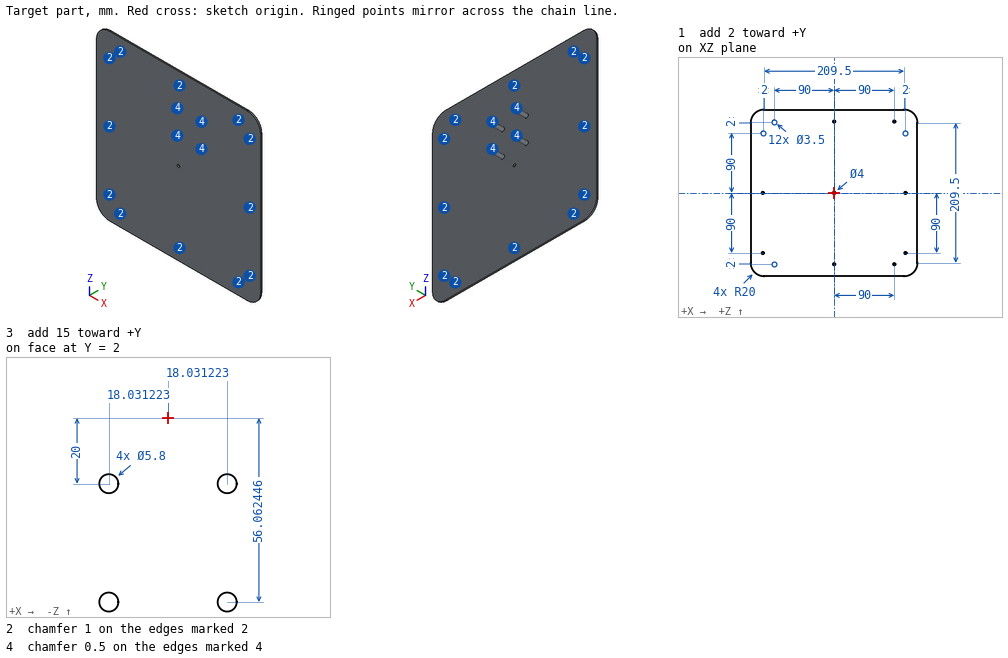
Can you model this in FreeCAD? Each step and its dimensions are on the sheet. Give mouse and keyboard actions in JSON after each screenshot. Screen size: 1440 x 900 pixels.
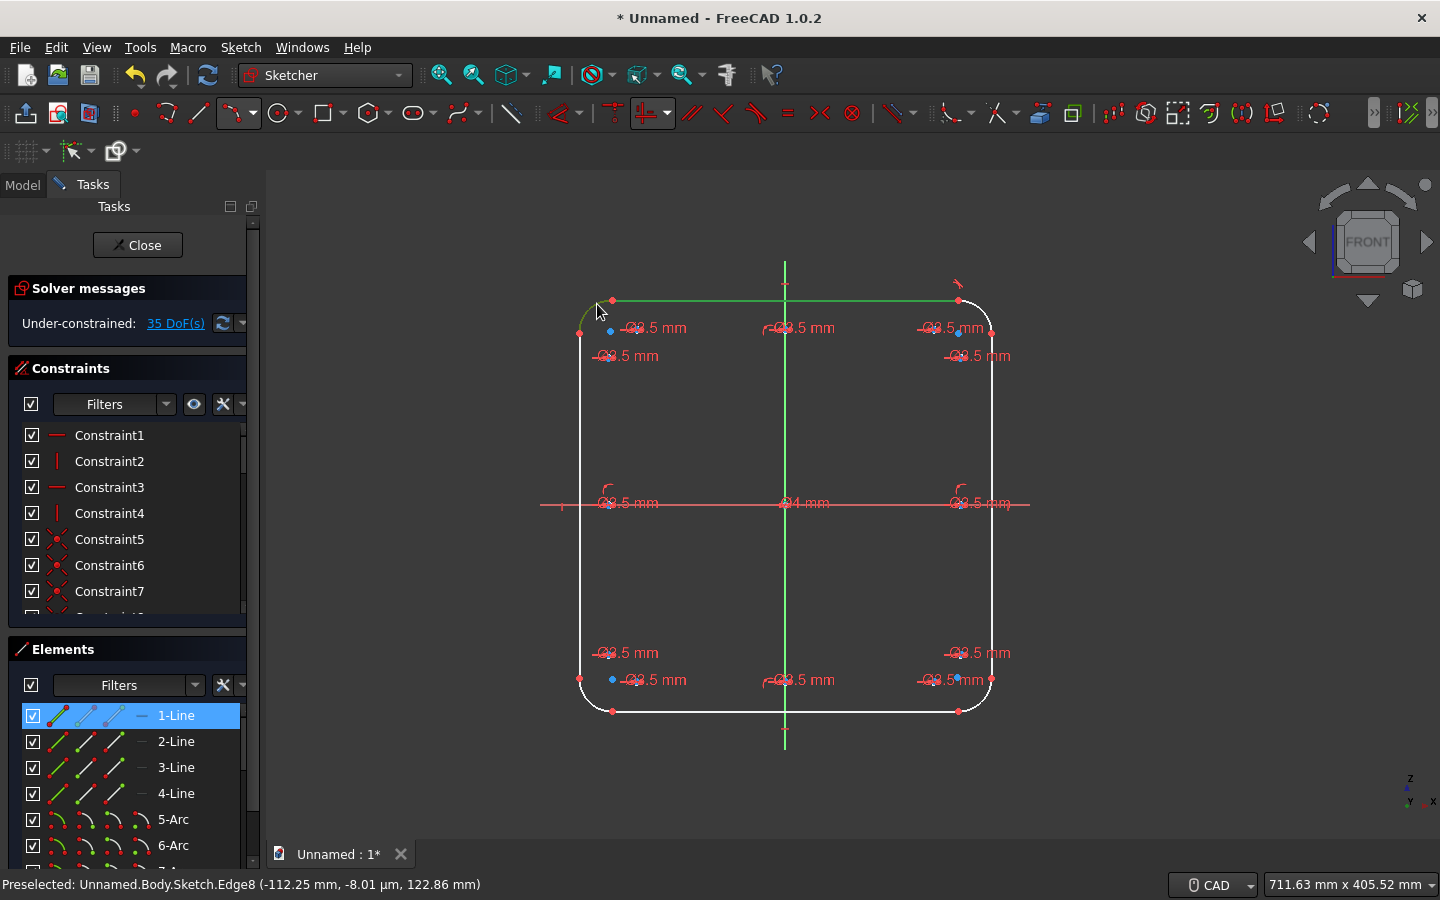
{"action": "key", "text": "t"}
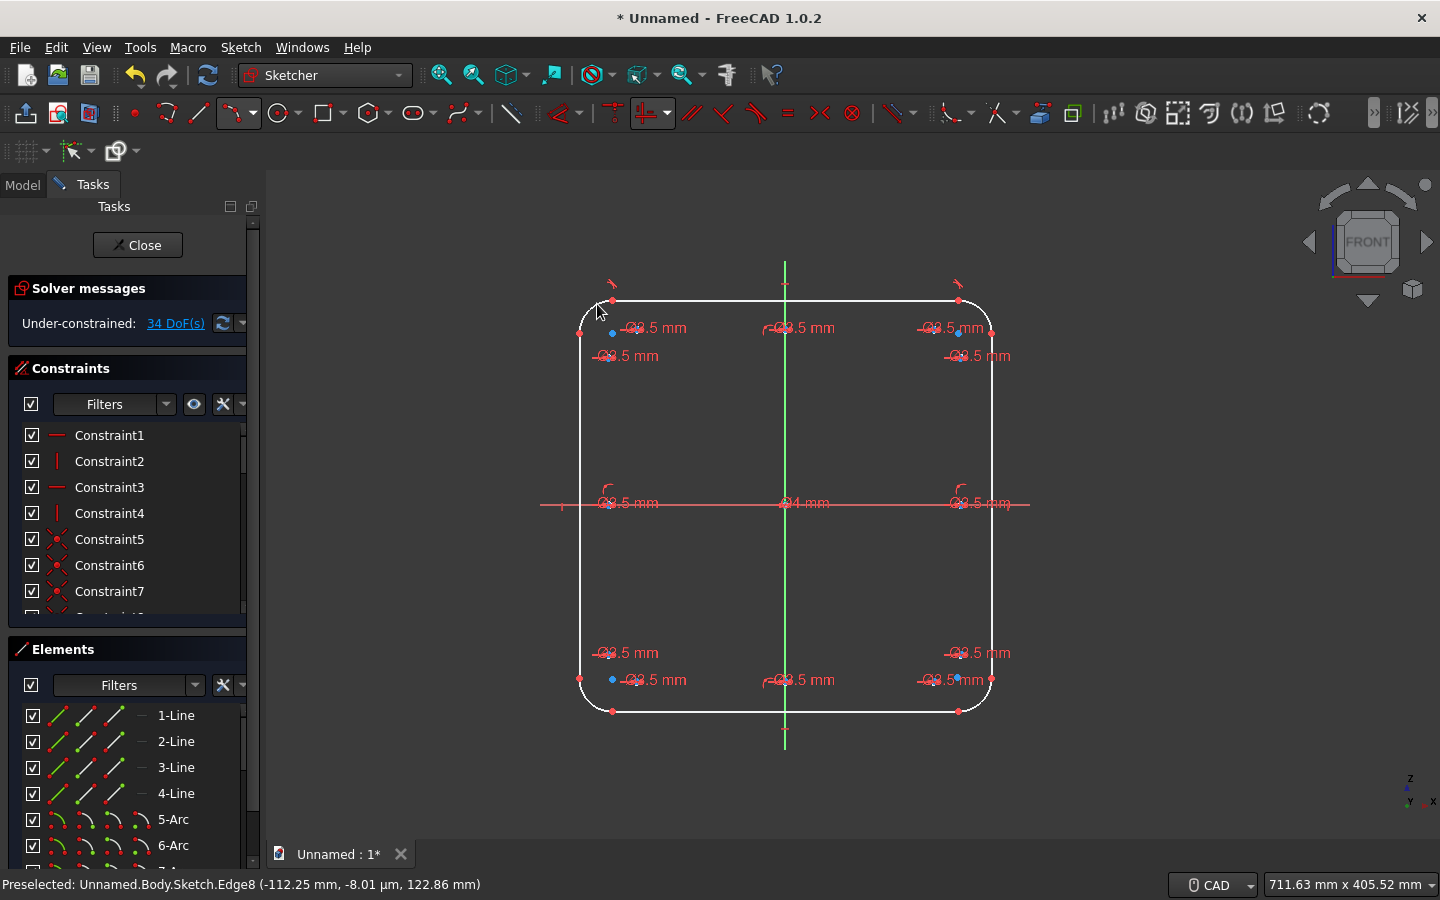
{"action": "left_click", "coordinate": [992, 437]}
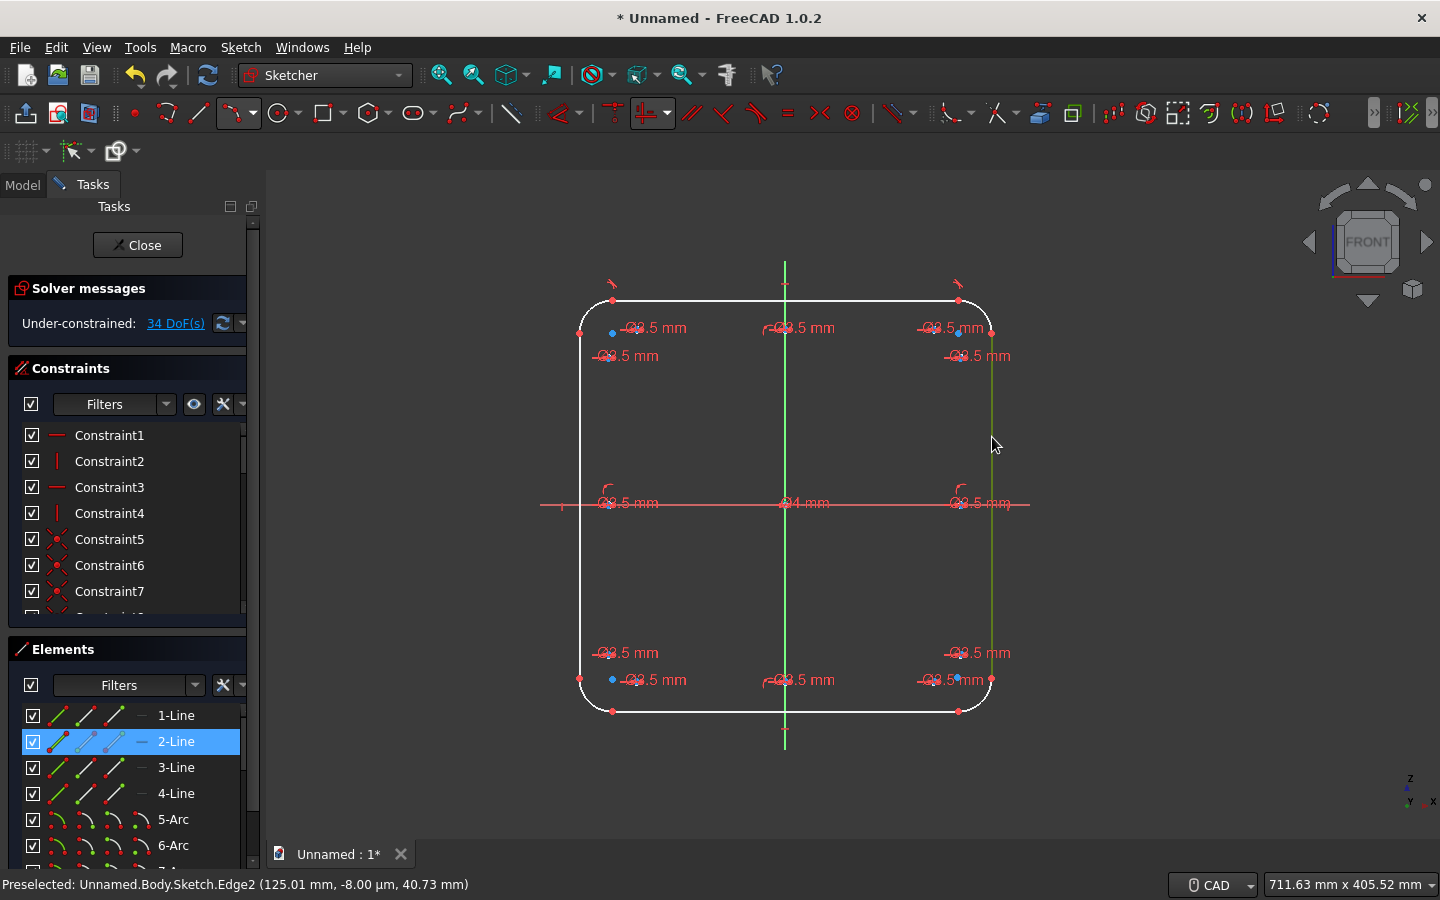
{"action": "left_click", "coordinate": [988, 319]}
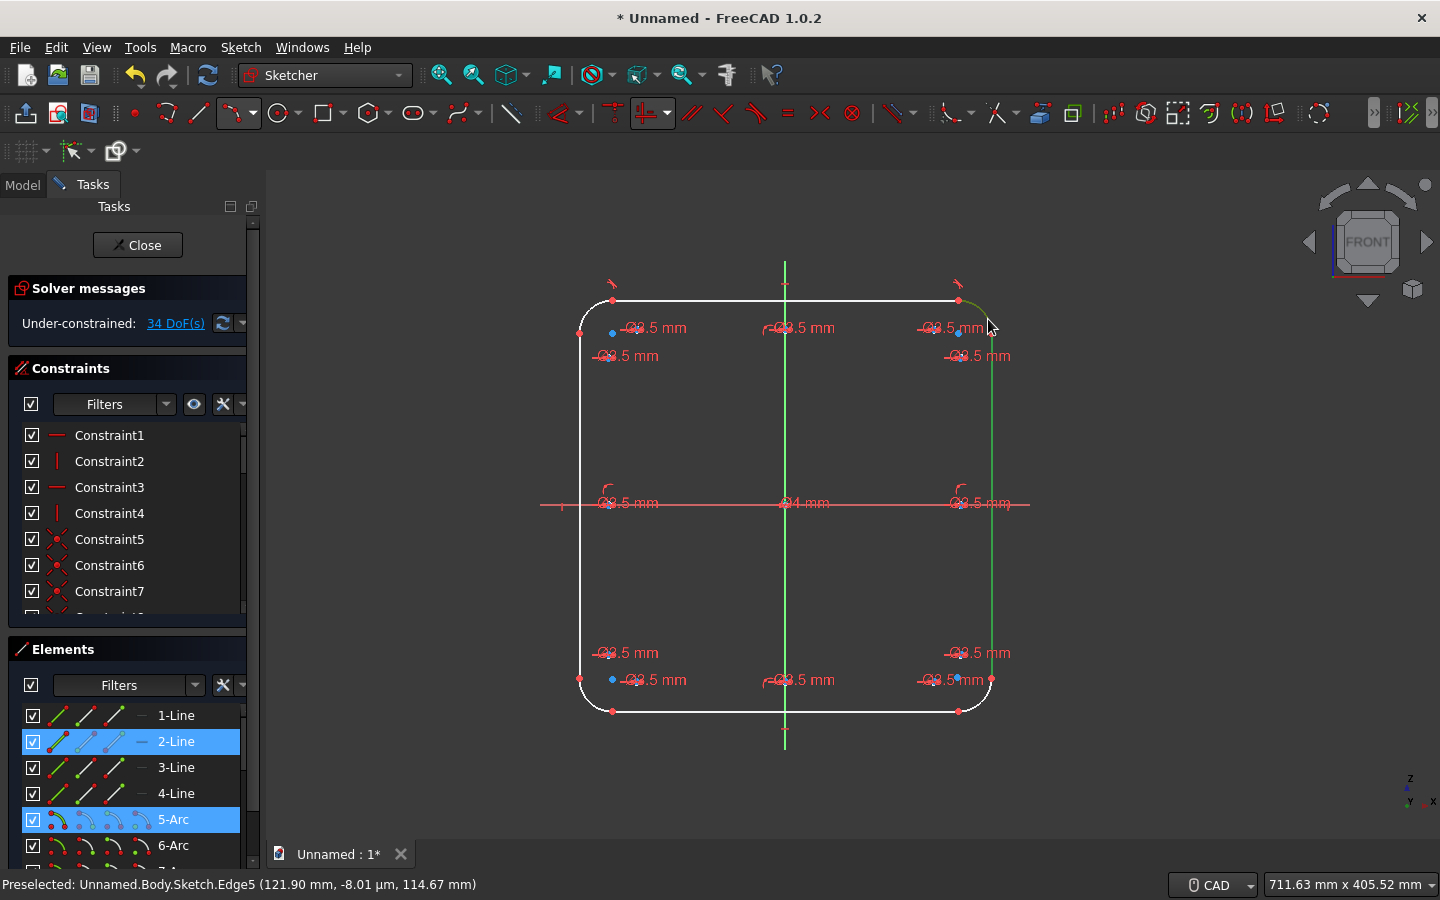
{"action": "left_click", "coordinate": [756, 114]}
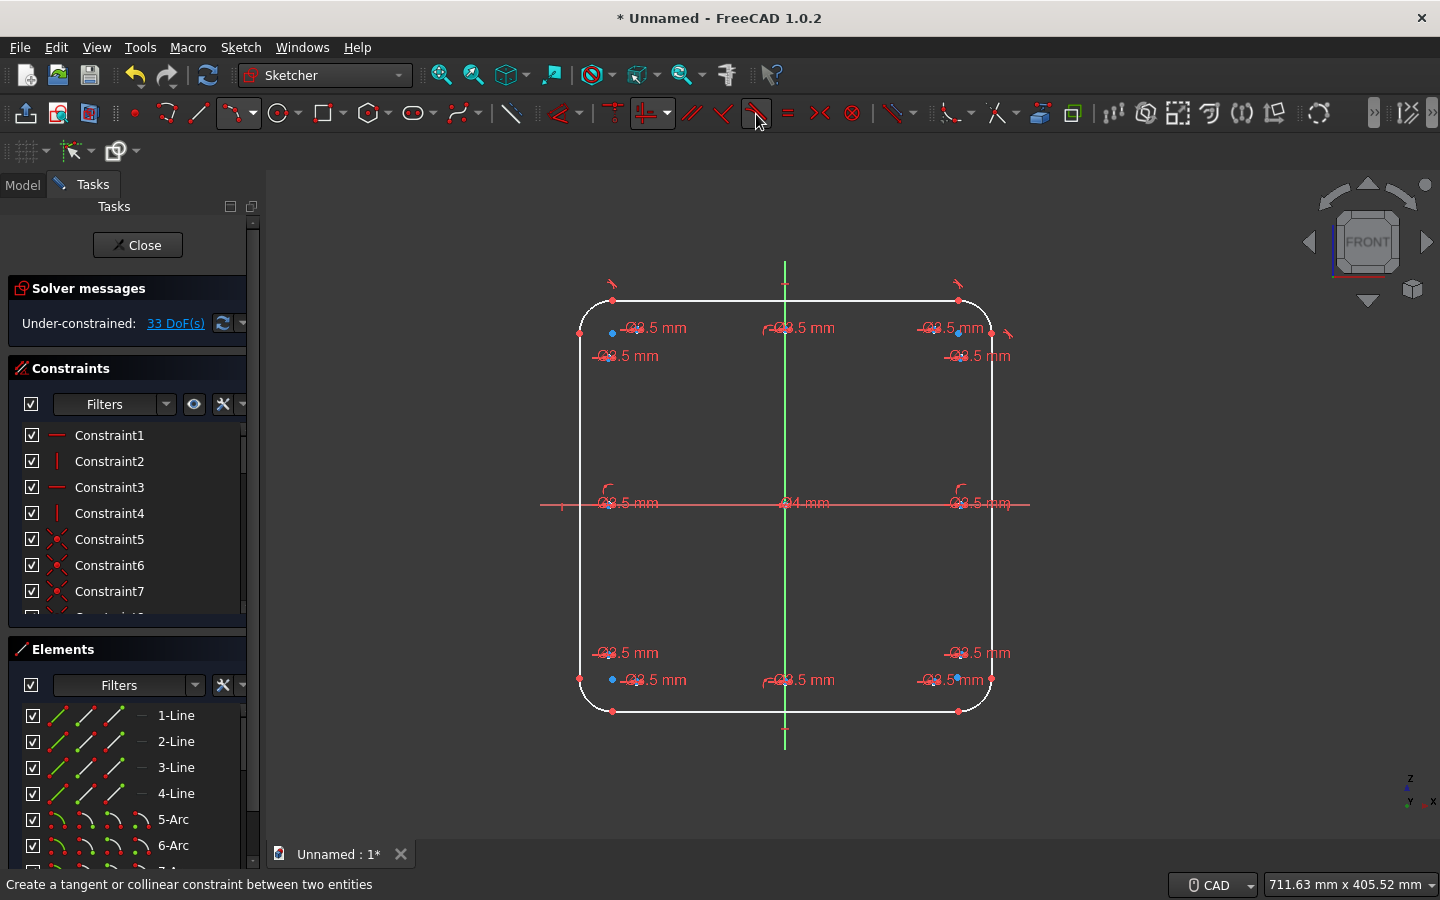
{"action": "left_click", "coordinate": [992, 437]}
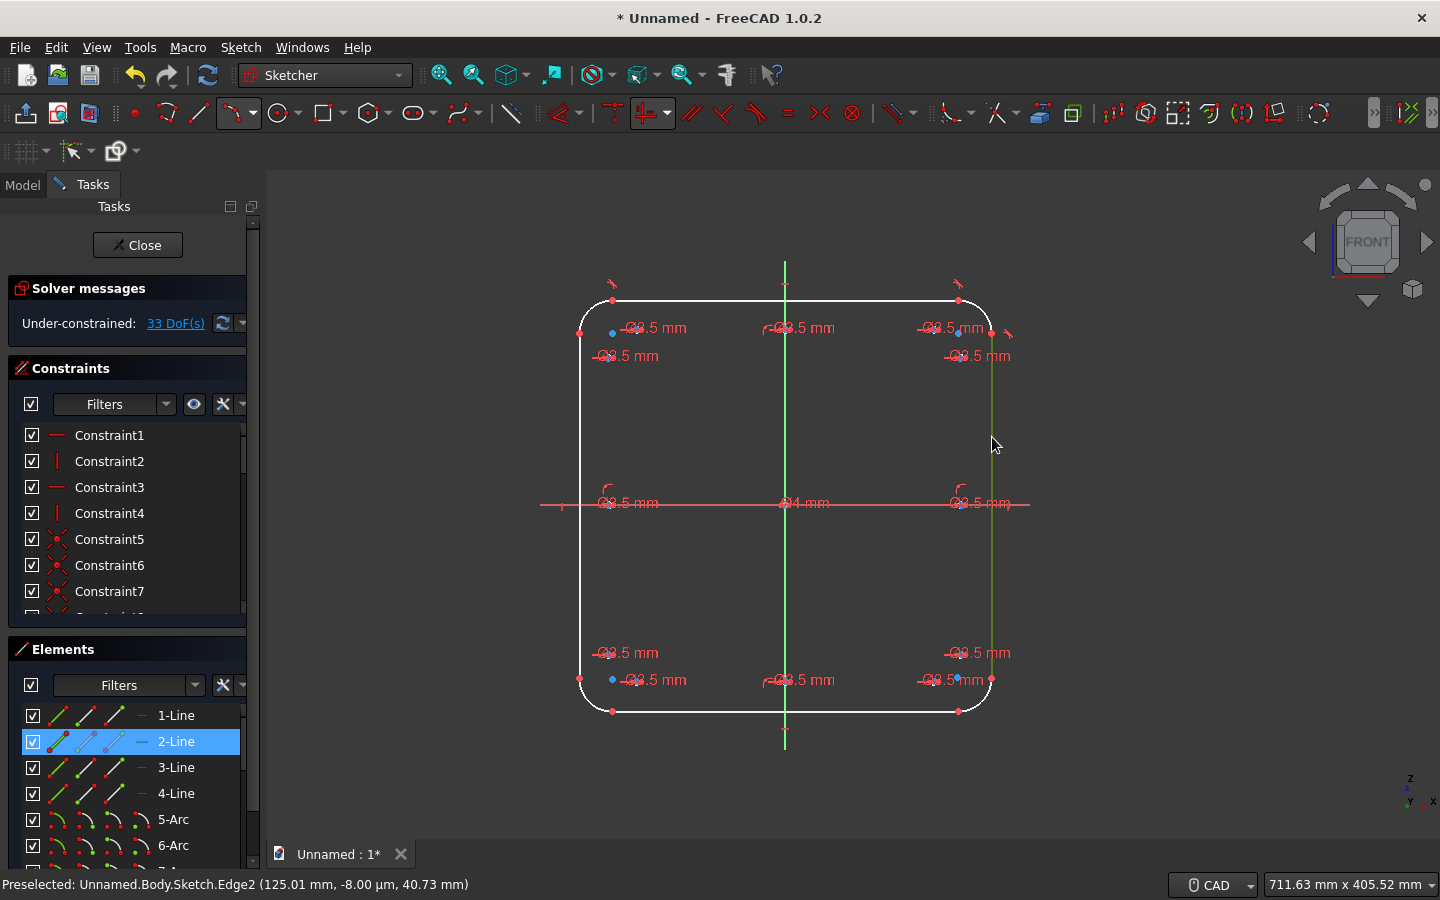
{"action": "left_click", "coordinate": [973, 708]}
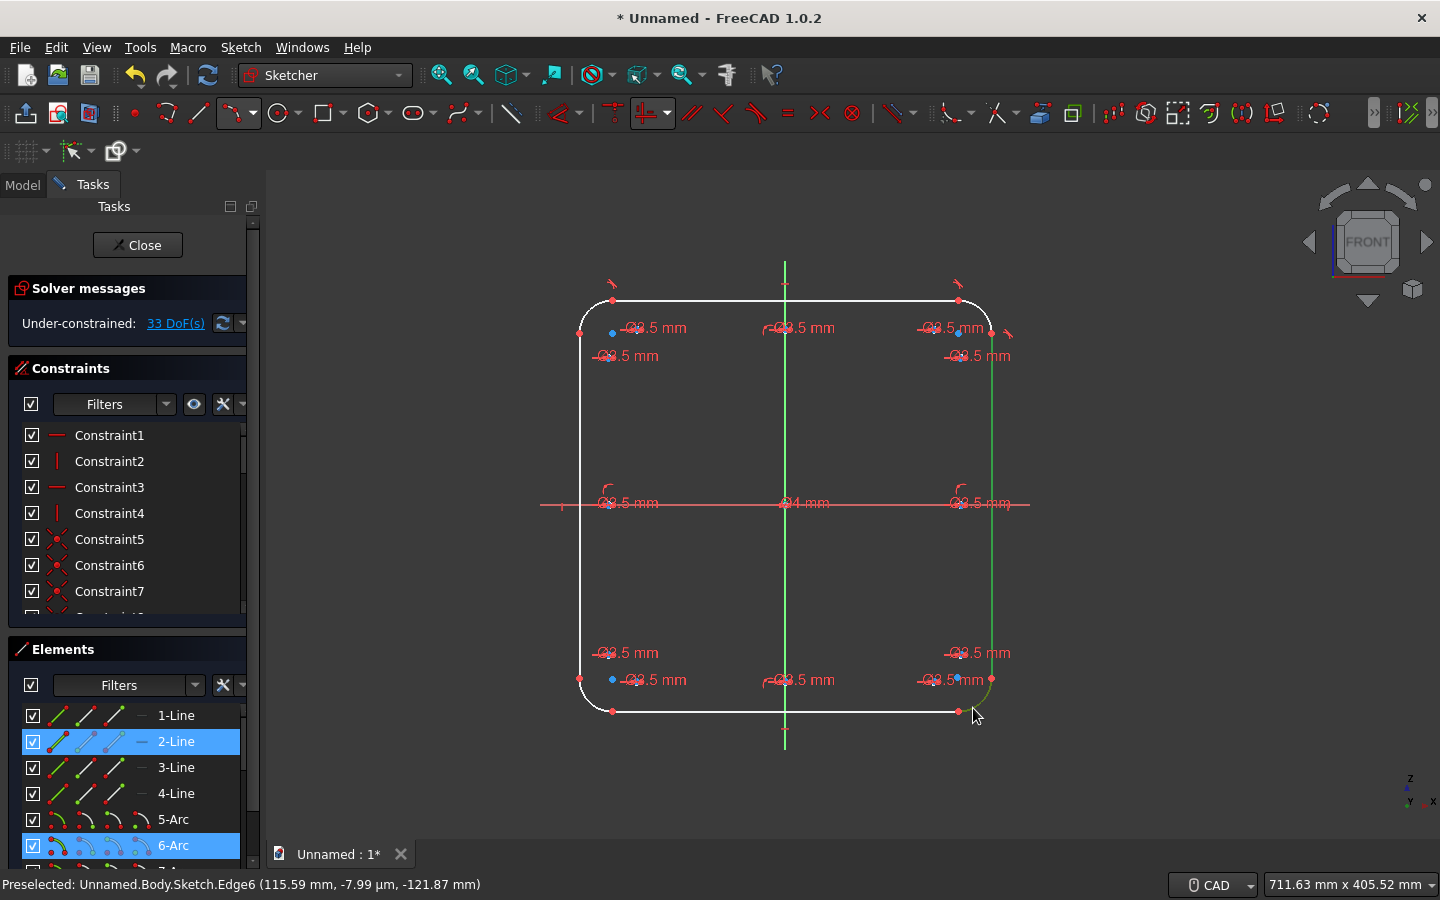
{"action": "key", "text": "t"}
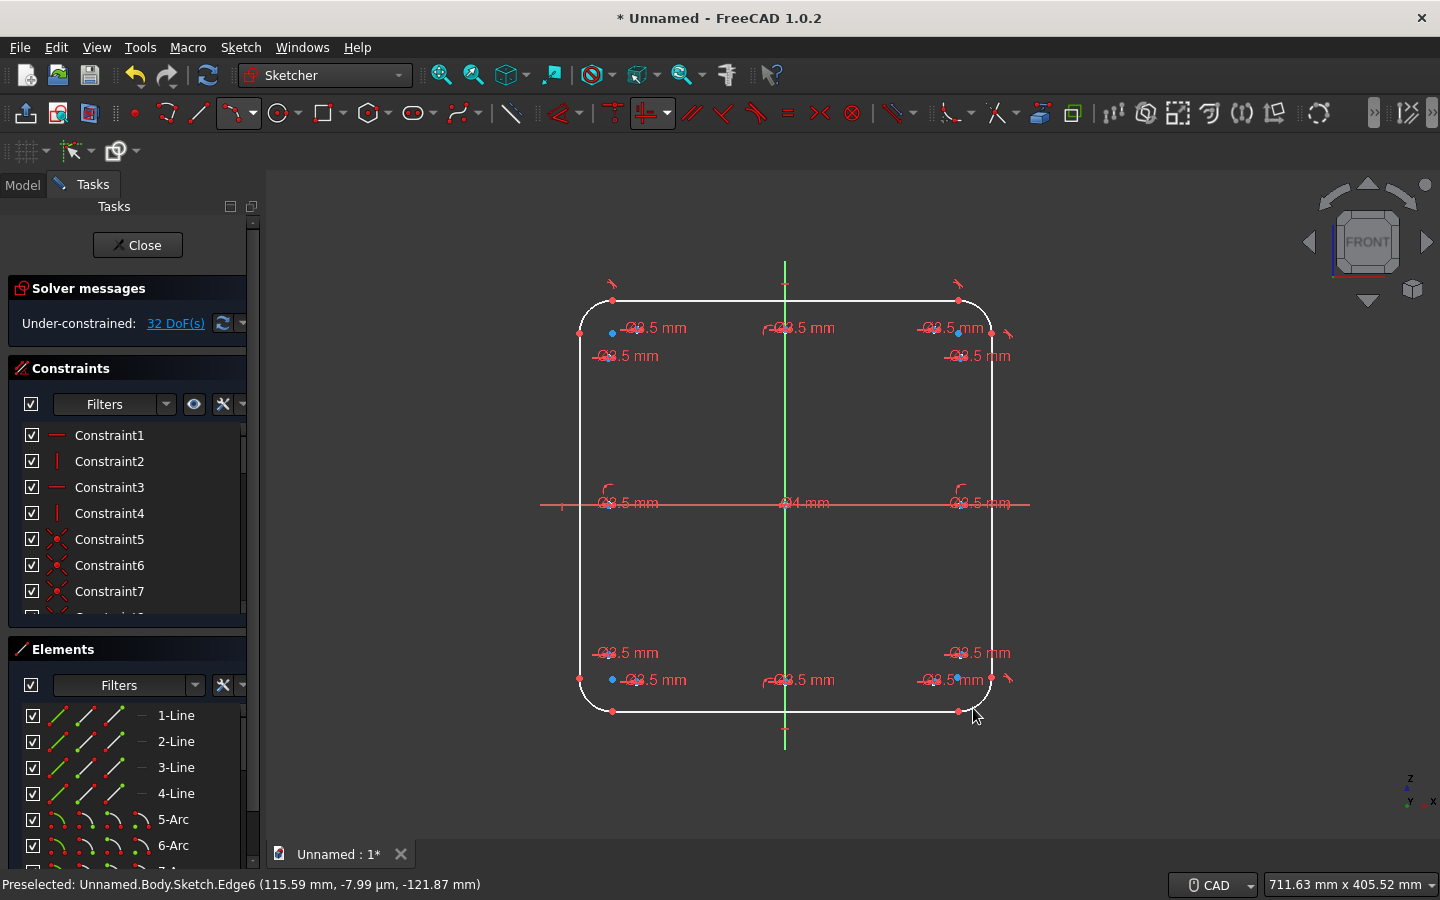
{"action": "left_click", "coordinate": [855, 712]}